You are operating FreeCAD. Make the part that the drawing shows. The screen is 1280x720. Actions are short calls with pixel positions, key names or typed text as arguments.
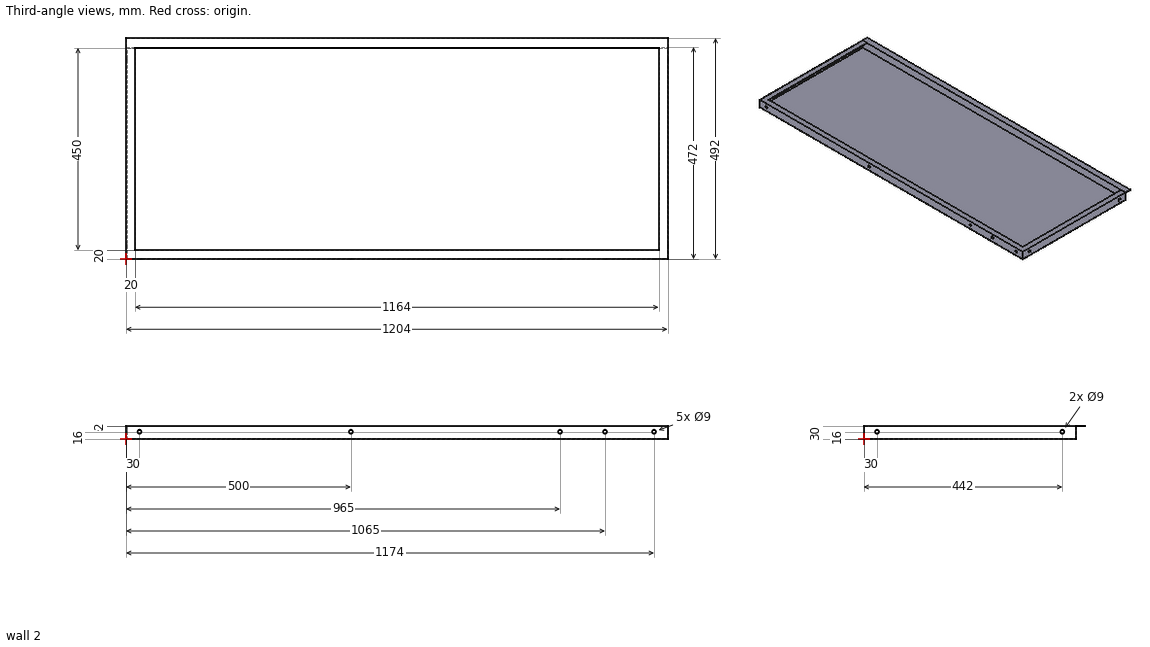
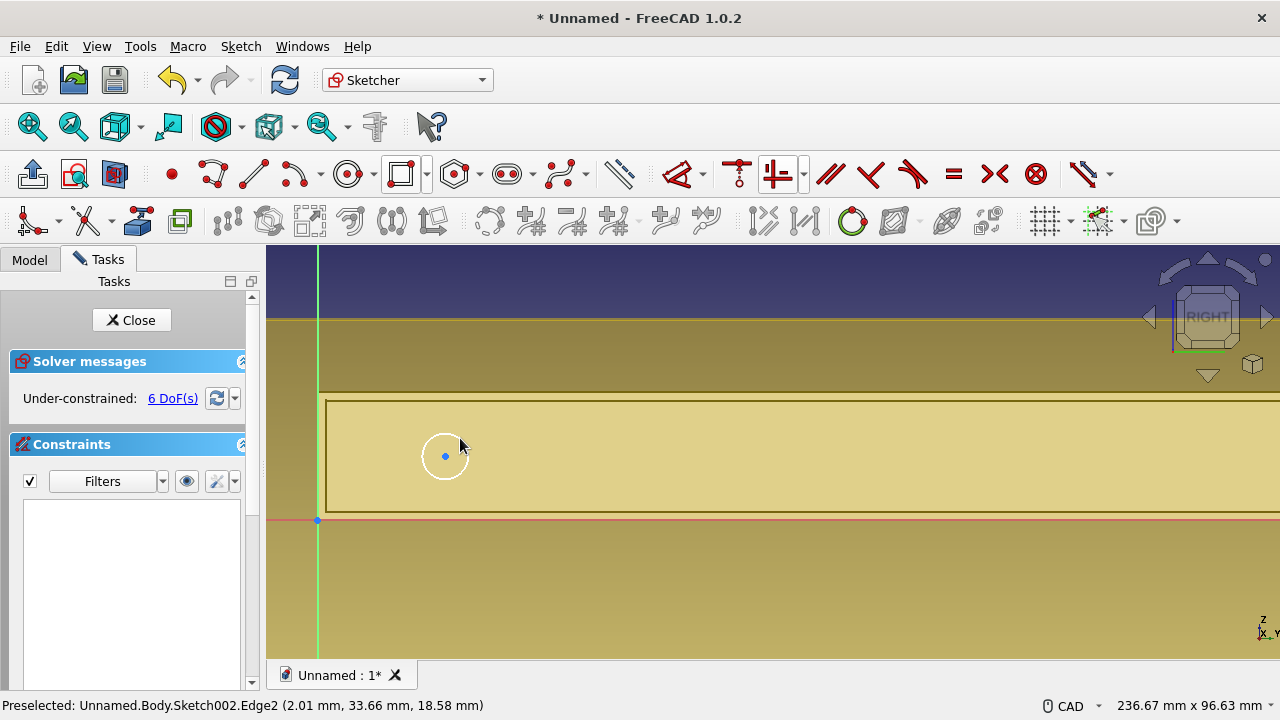
scroll(459, 441, down, 6)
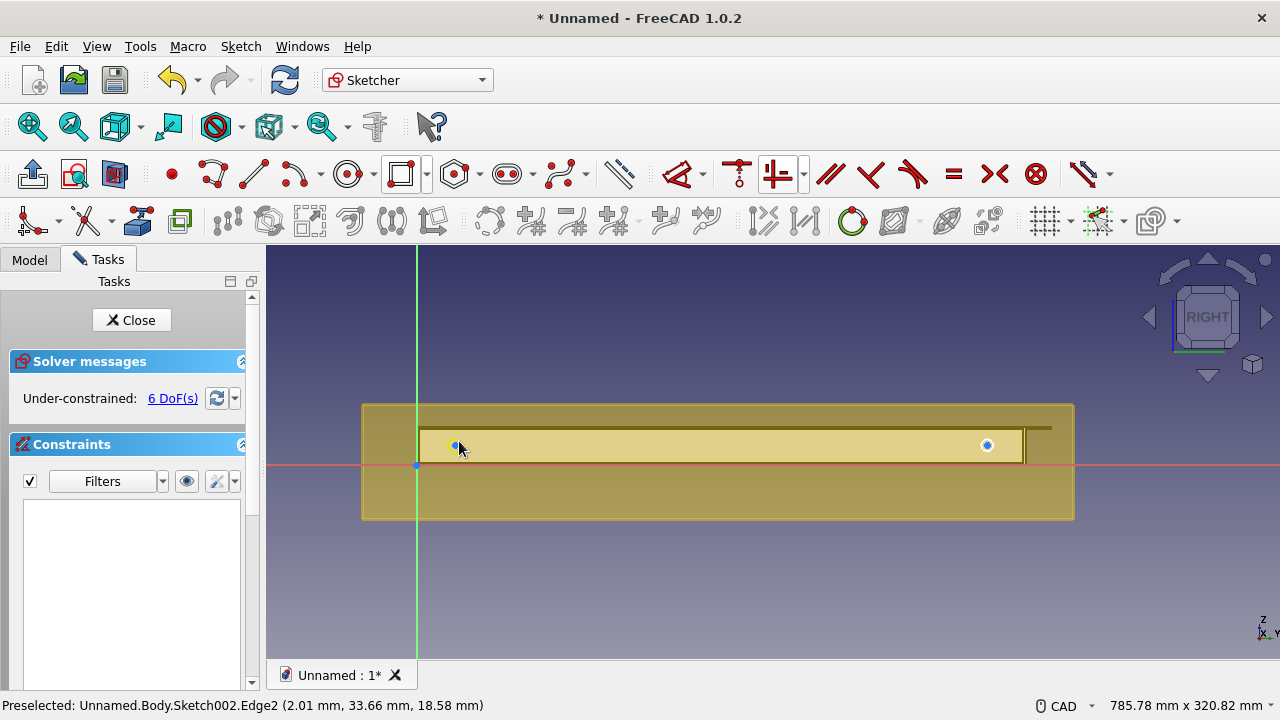
scroll(991, 441, up, 5)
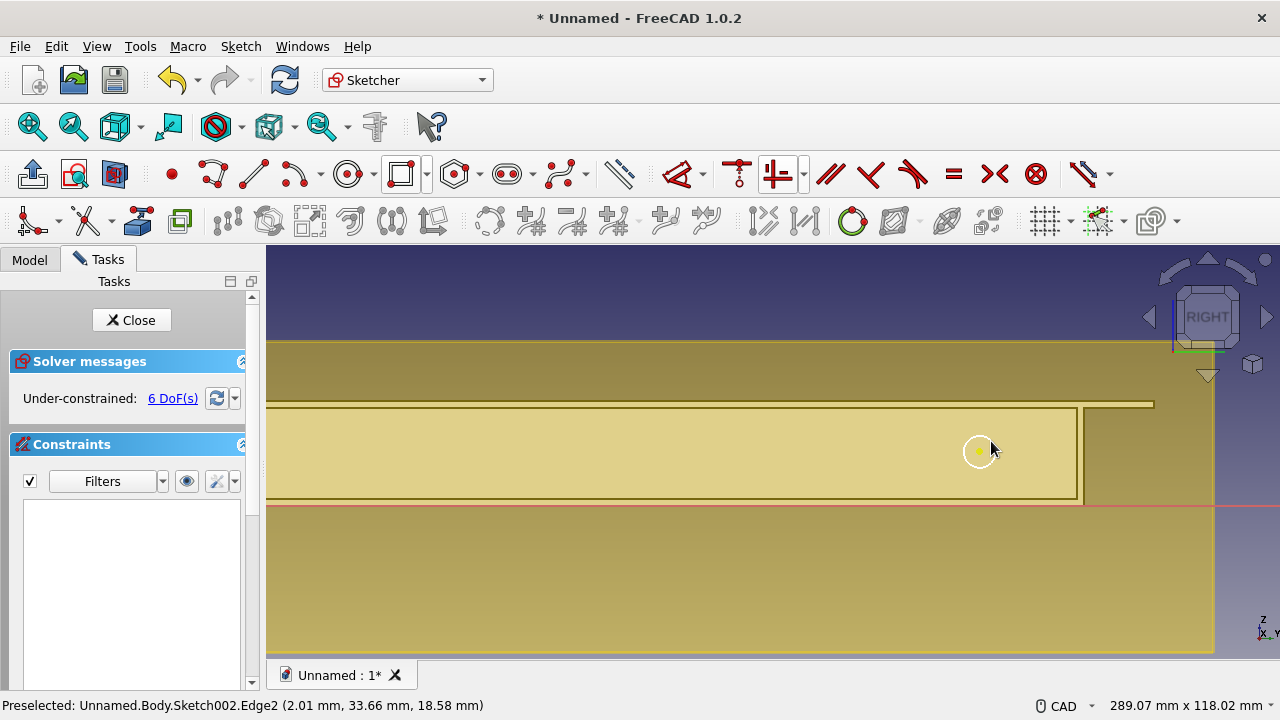
click(991, 441)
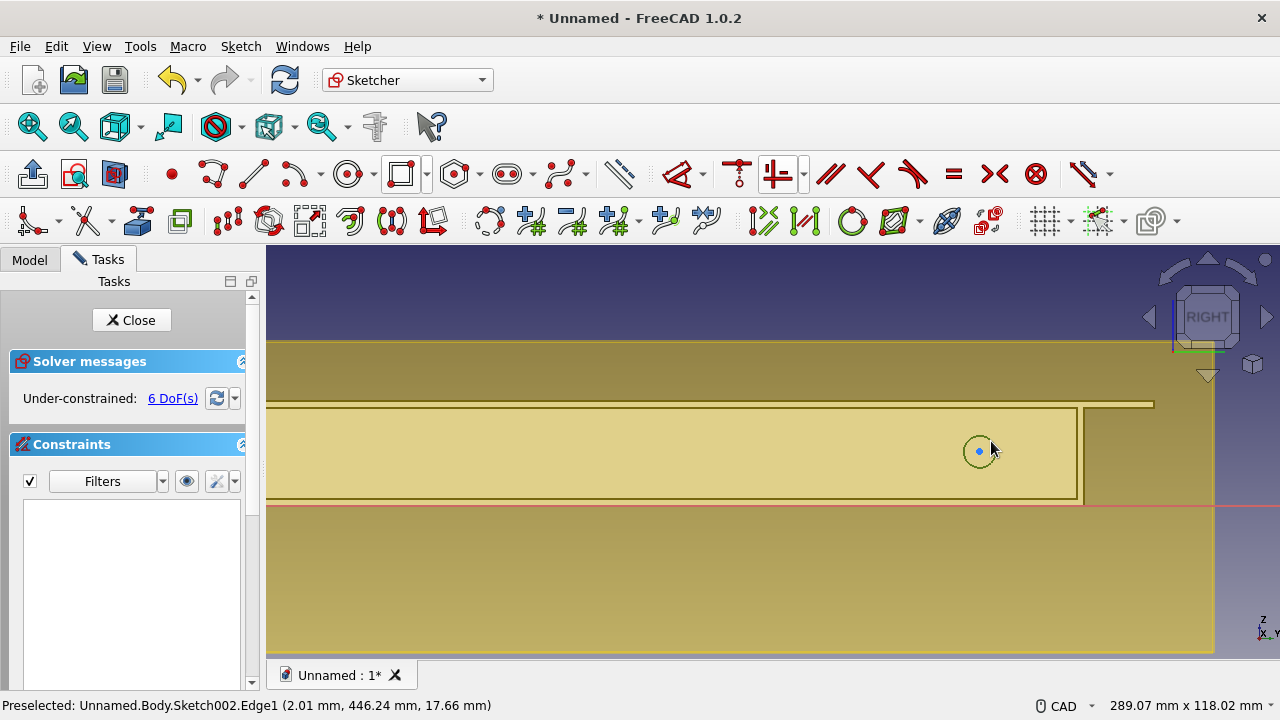
scroll(991, 441, down, 5)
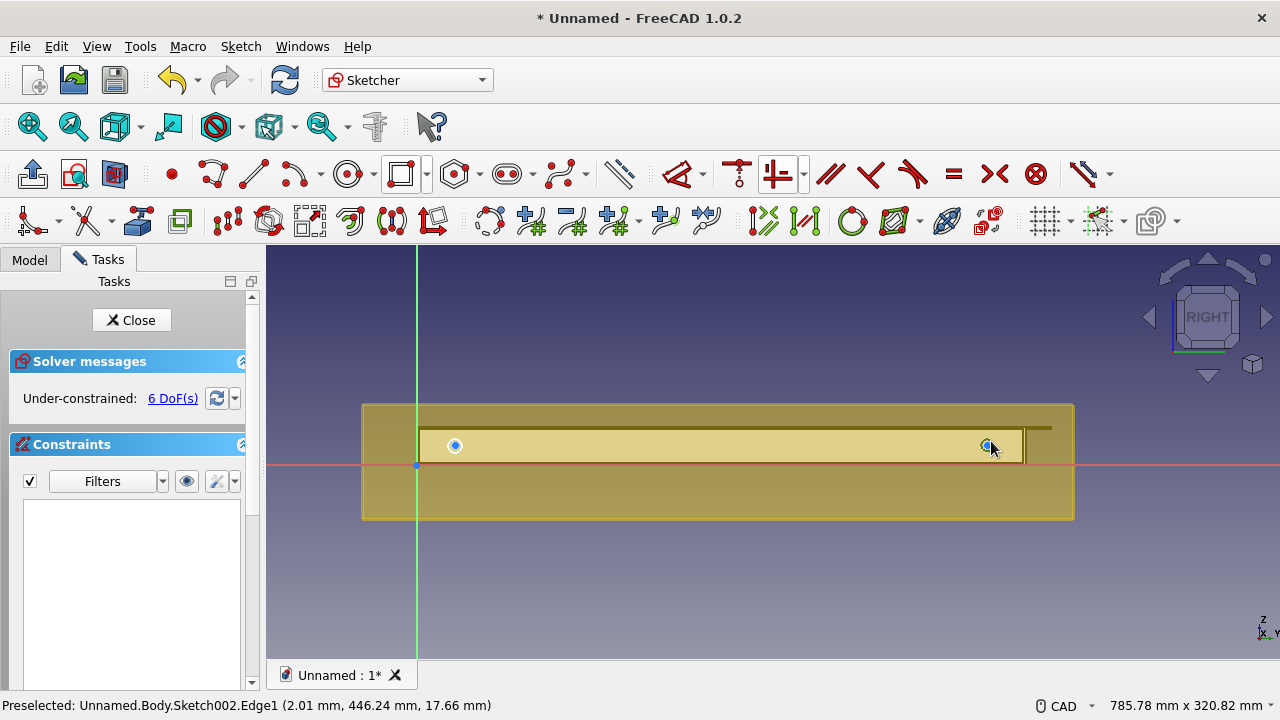
scroll(460, 441, up, 4)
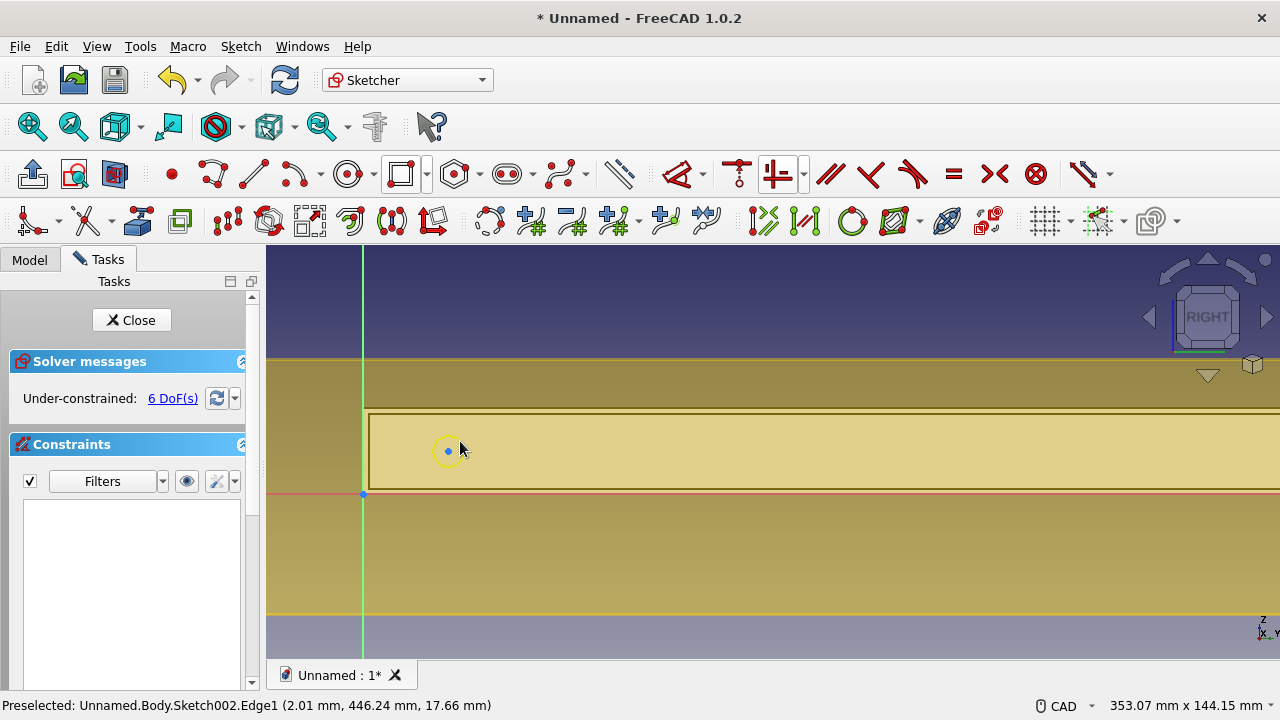
click(459, 441)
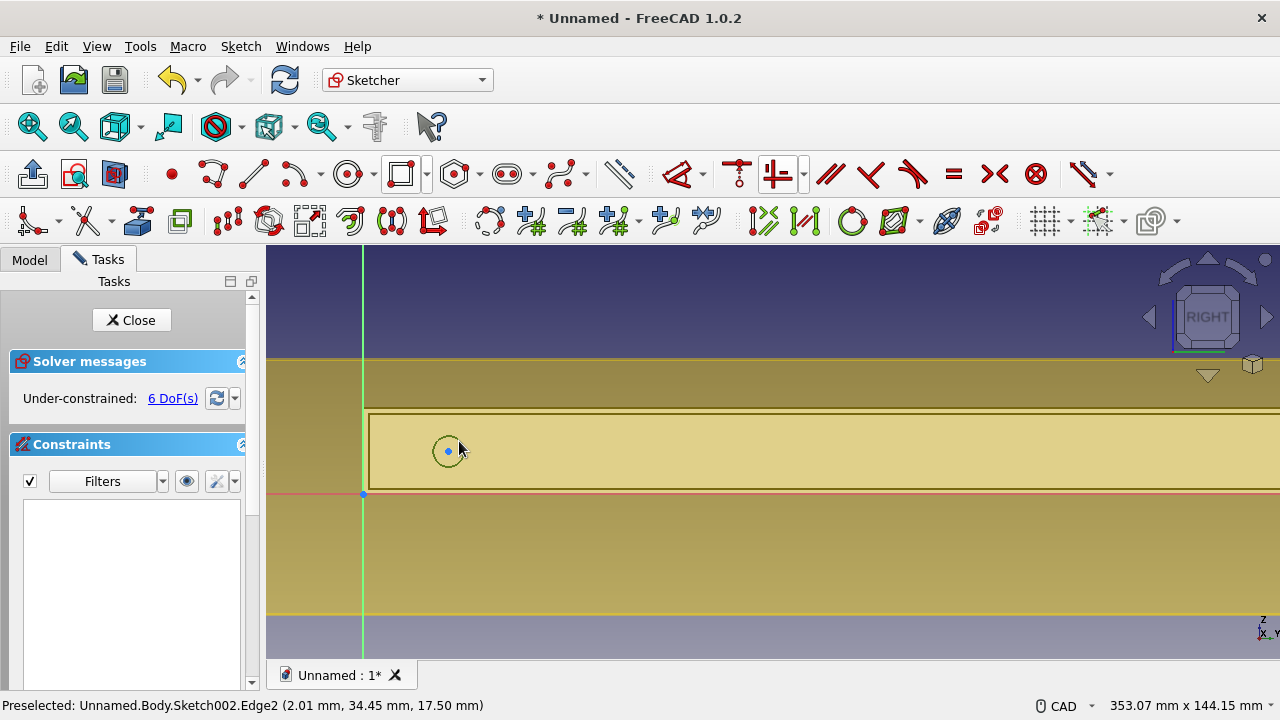
click(954, 174)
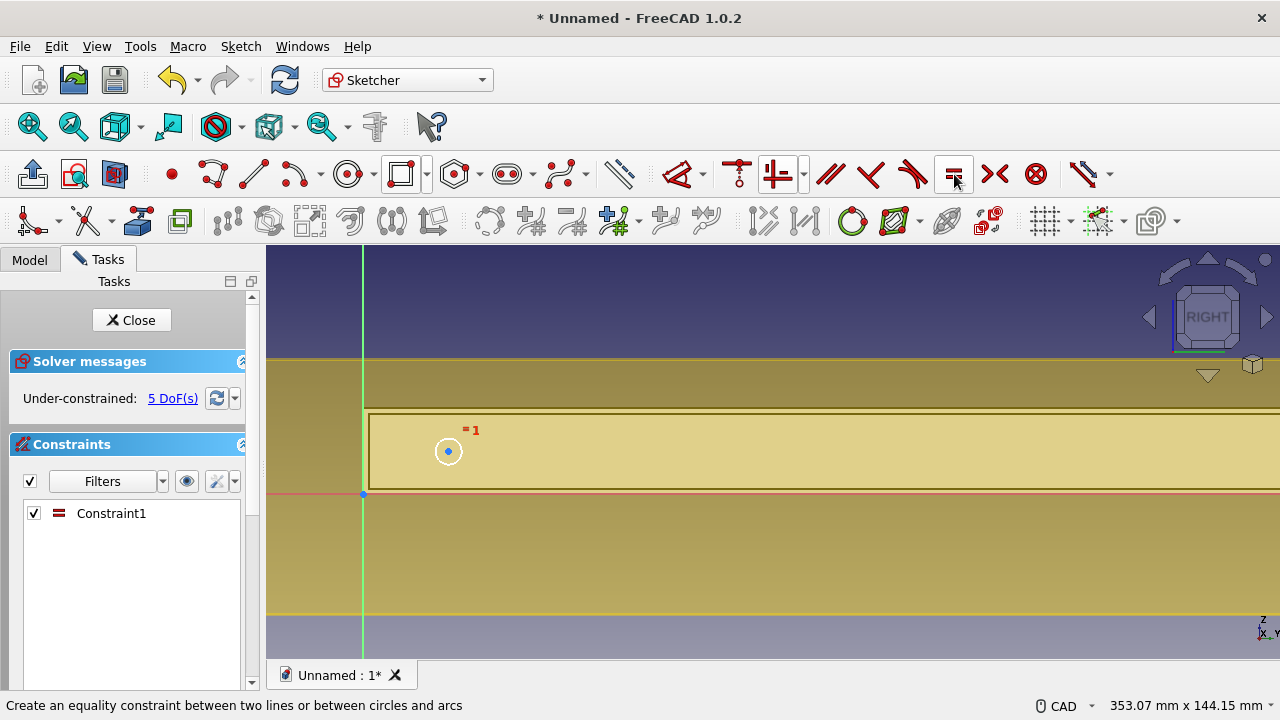
click(676, 174)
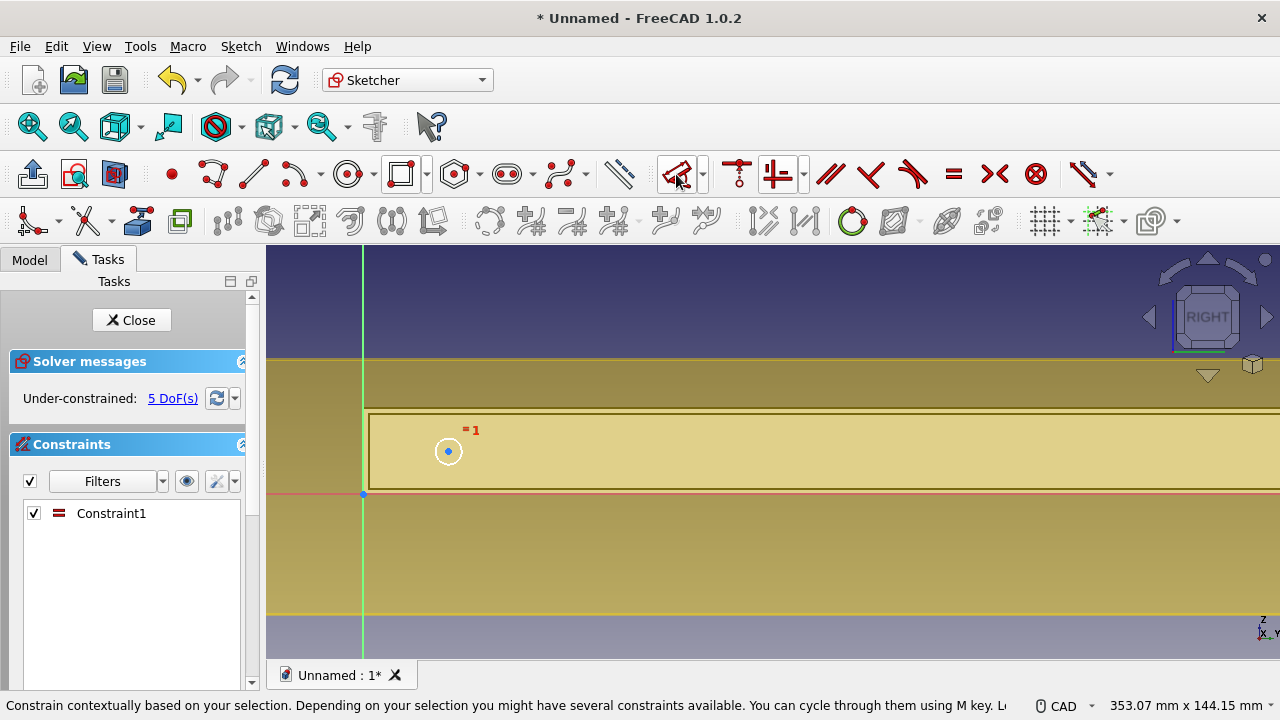
scroll(460, 441, down, 4)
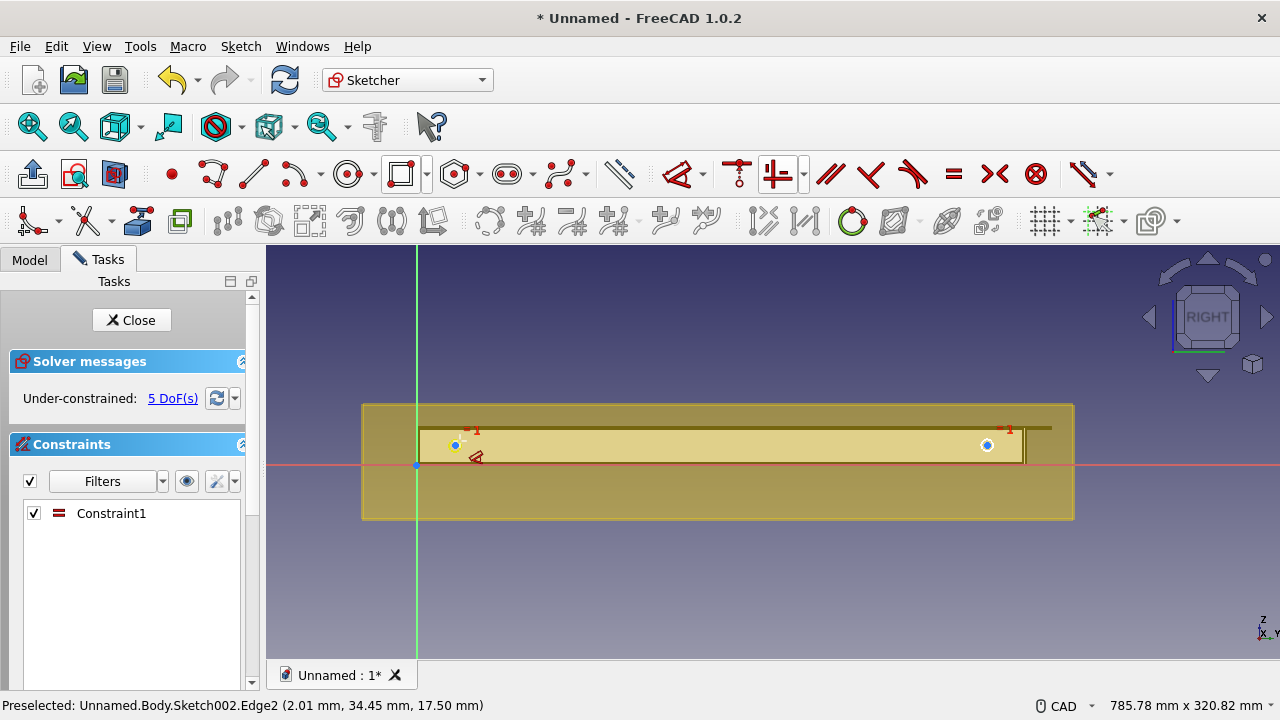
scroll(991, 441, up, 7)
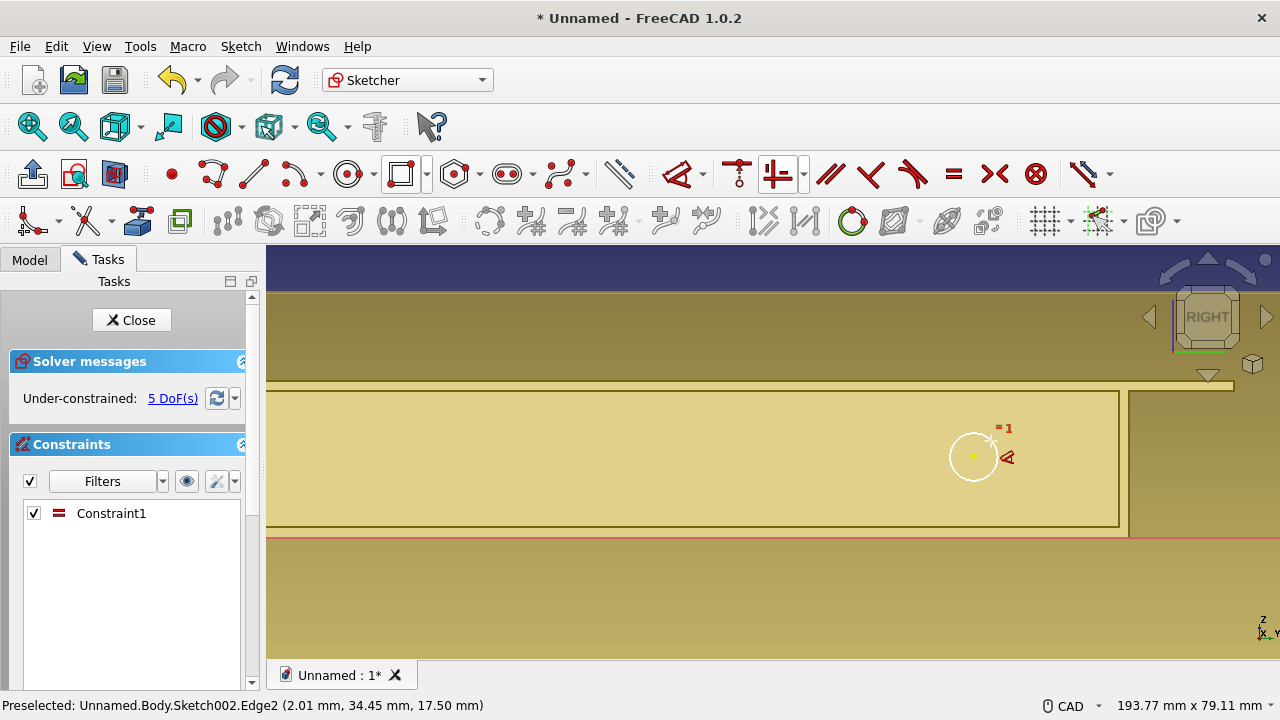
click(991, 440)
click(1014, 418)